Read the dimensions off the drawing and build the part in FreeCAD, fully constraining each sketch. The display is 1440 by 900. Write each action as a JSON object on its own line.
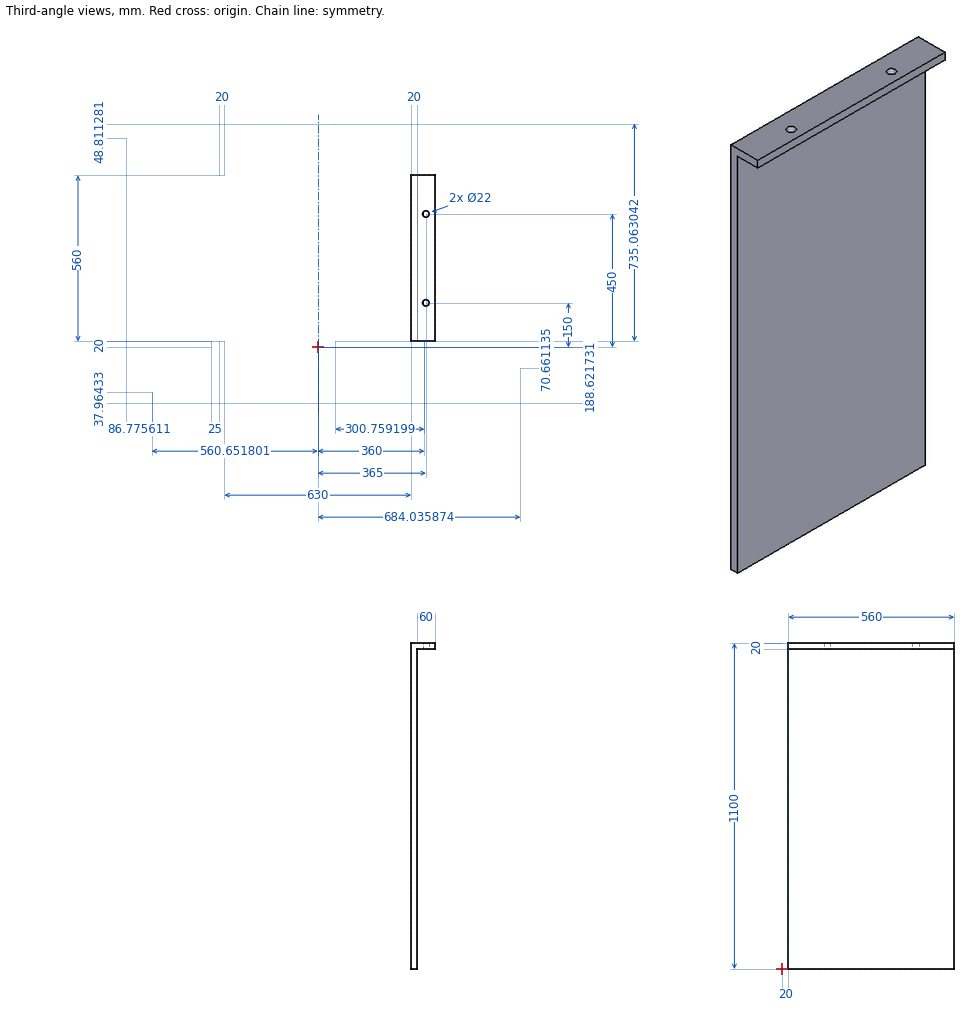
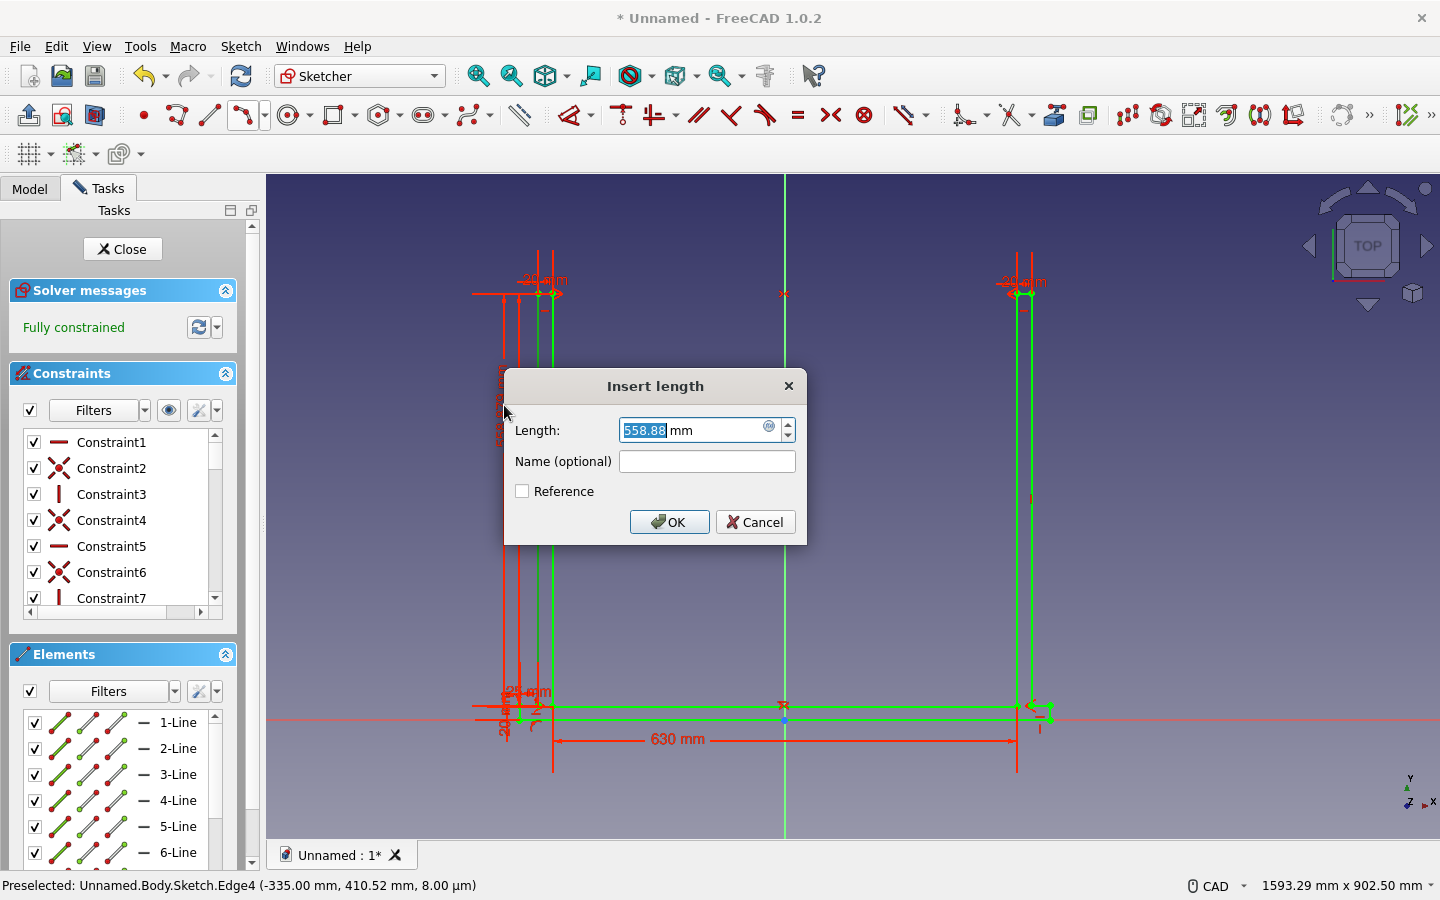
{"action": "type", "text": "560"}
{"action": "key", "text": "Return"}
{"action": "key", "text": "Escape"}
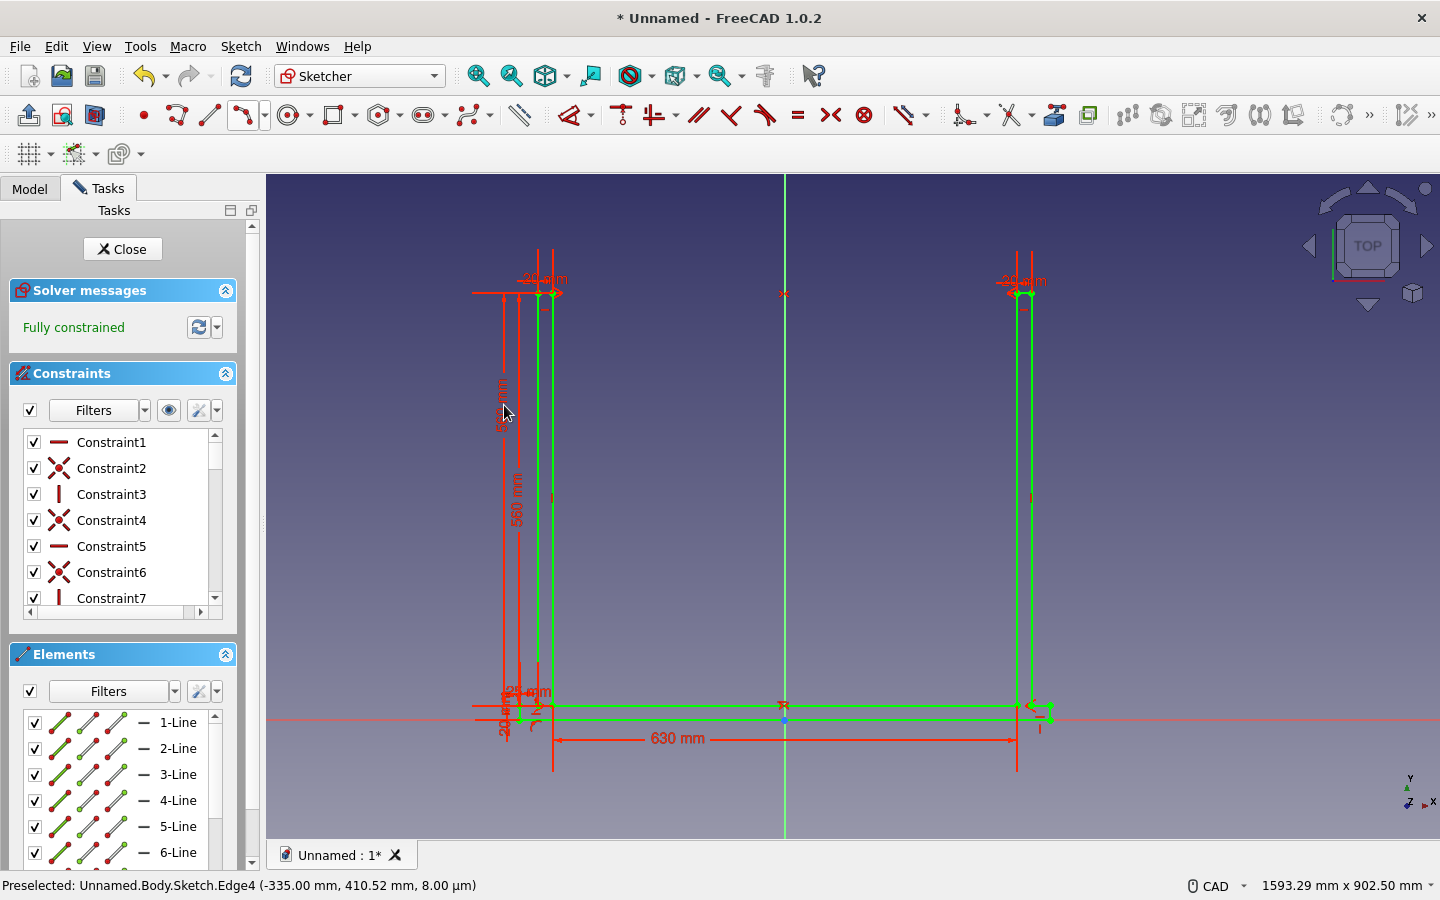
{"action": "left_click", "coordinate": [123, 249]}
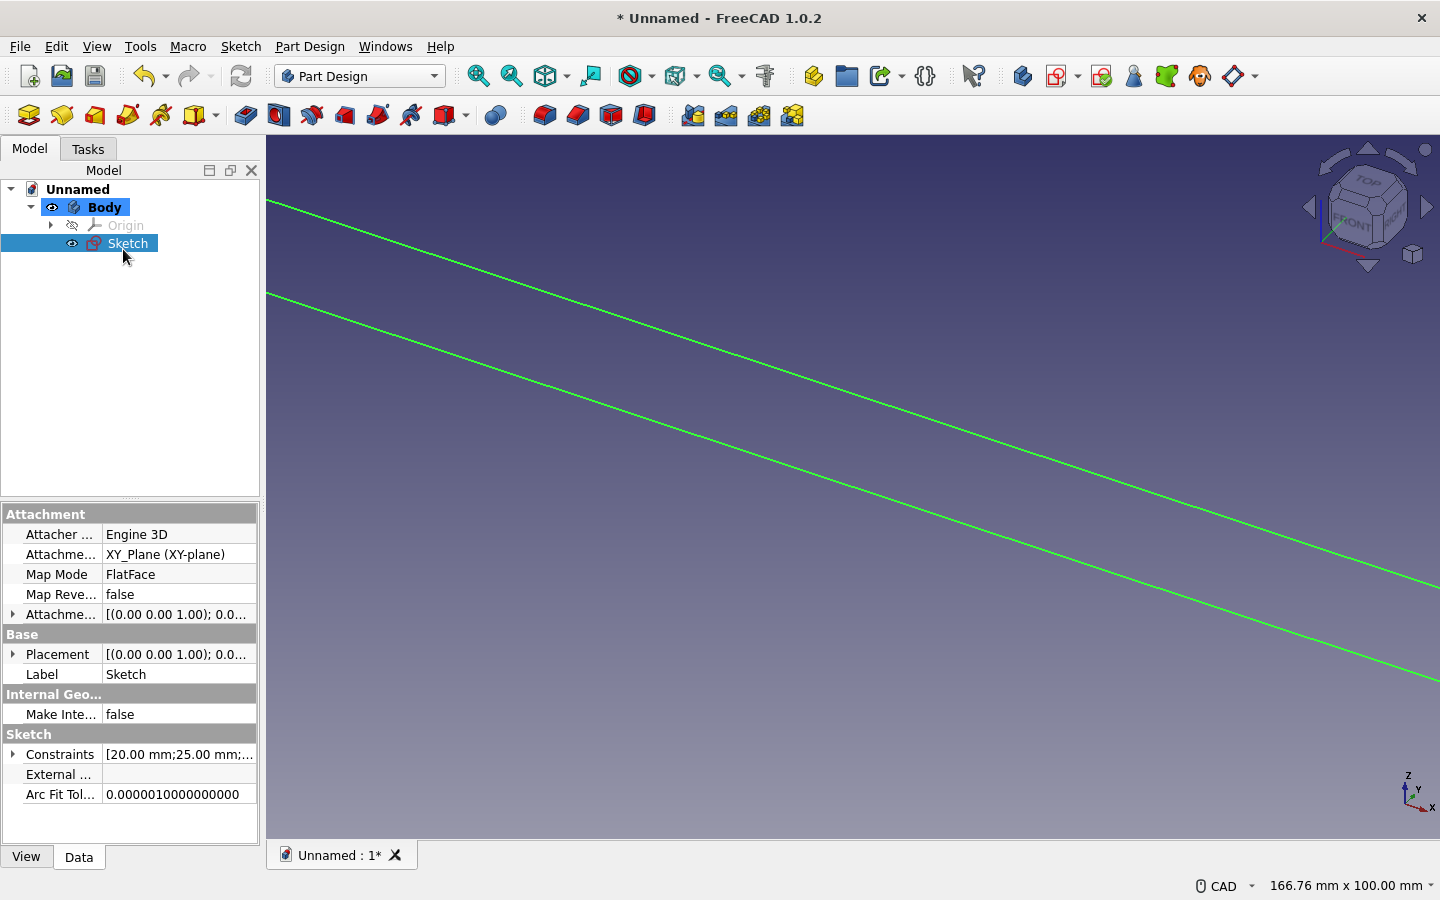
{"action": "left_click", "coordinate": [29, 116]}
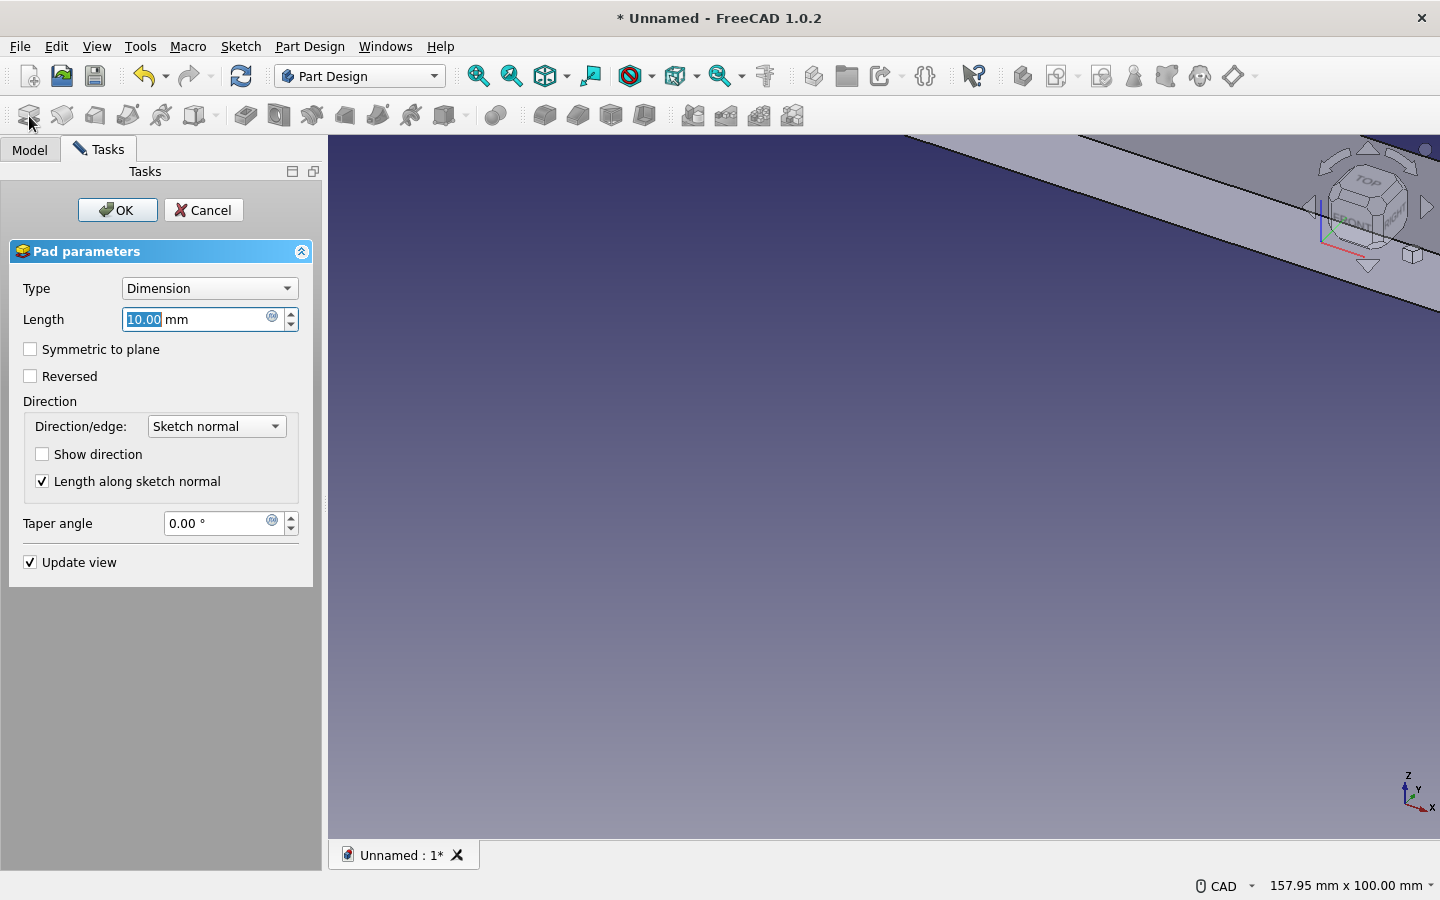
{"action": "type", "text": "1100"}
{"action": "key", "text": "Tab"}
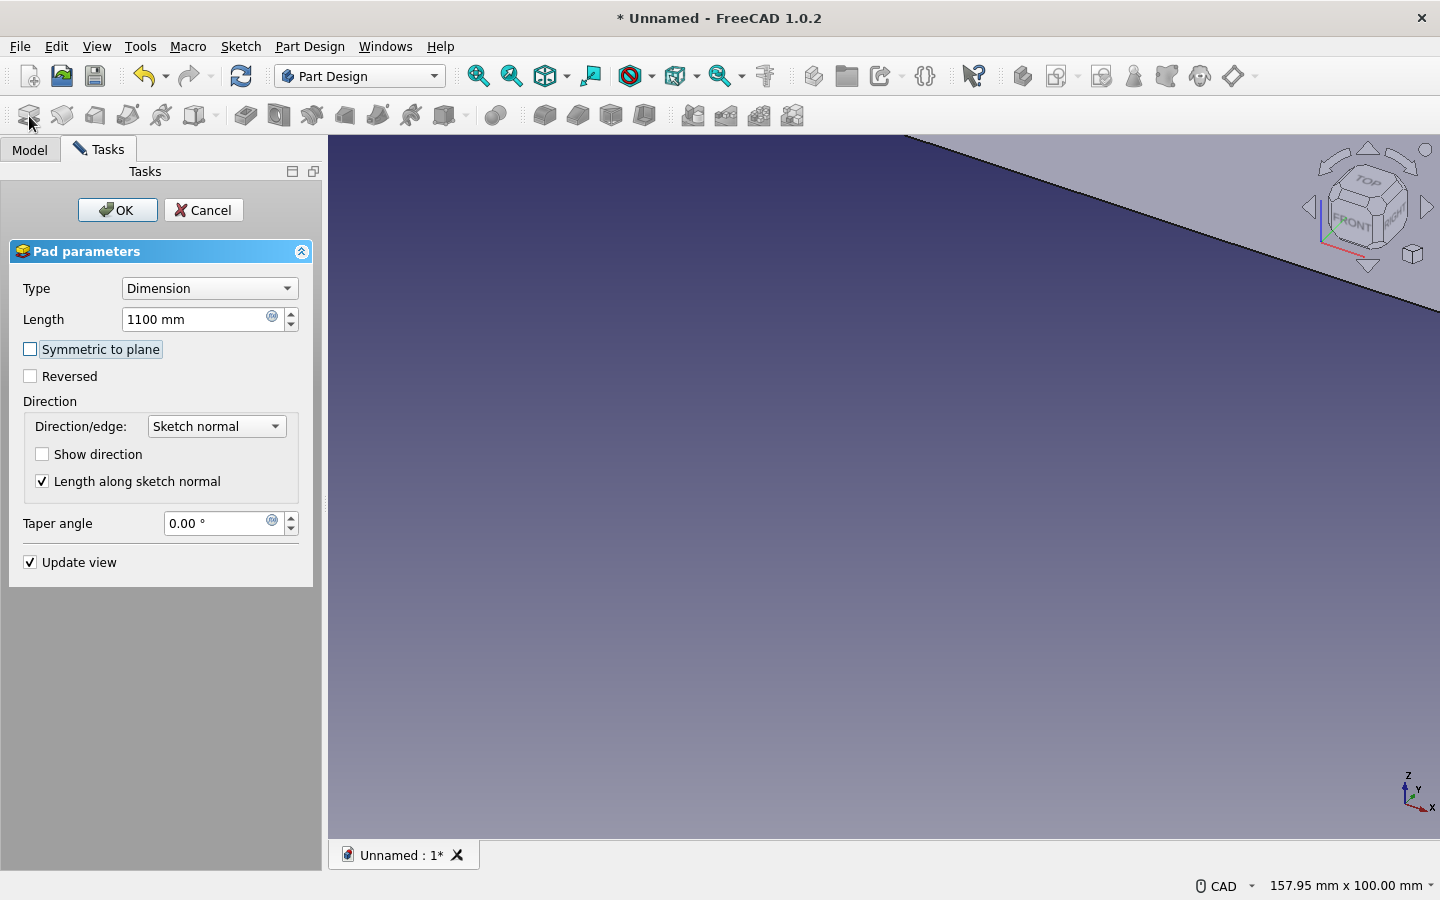
{"action": "left_click", "coordinate": [118, 210]}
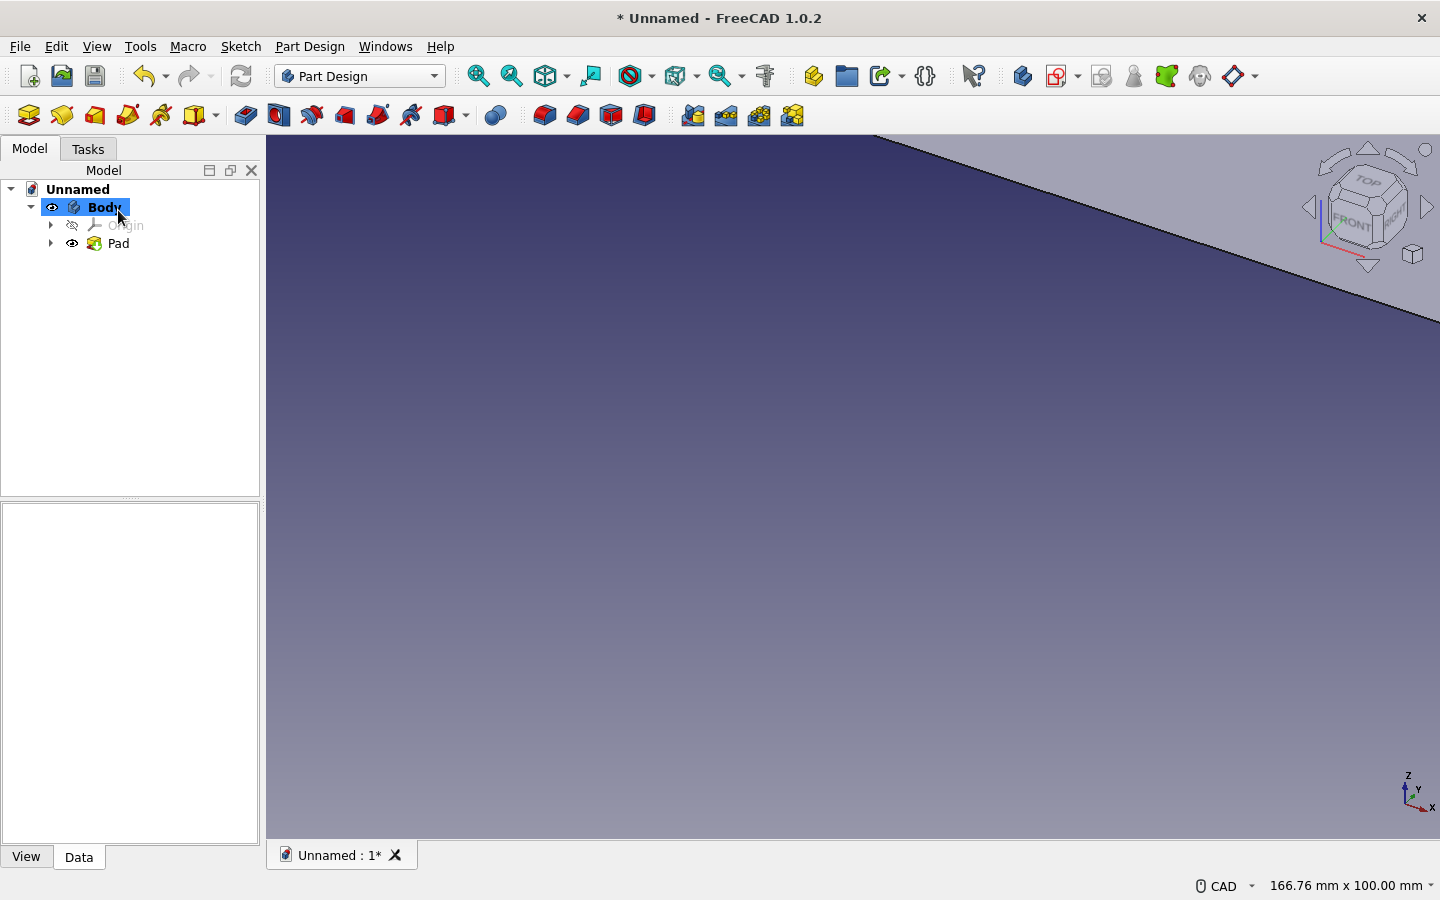
{"action": "left_click", "coordinate": [479, 76]}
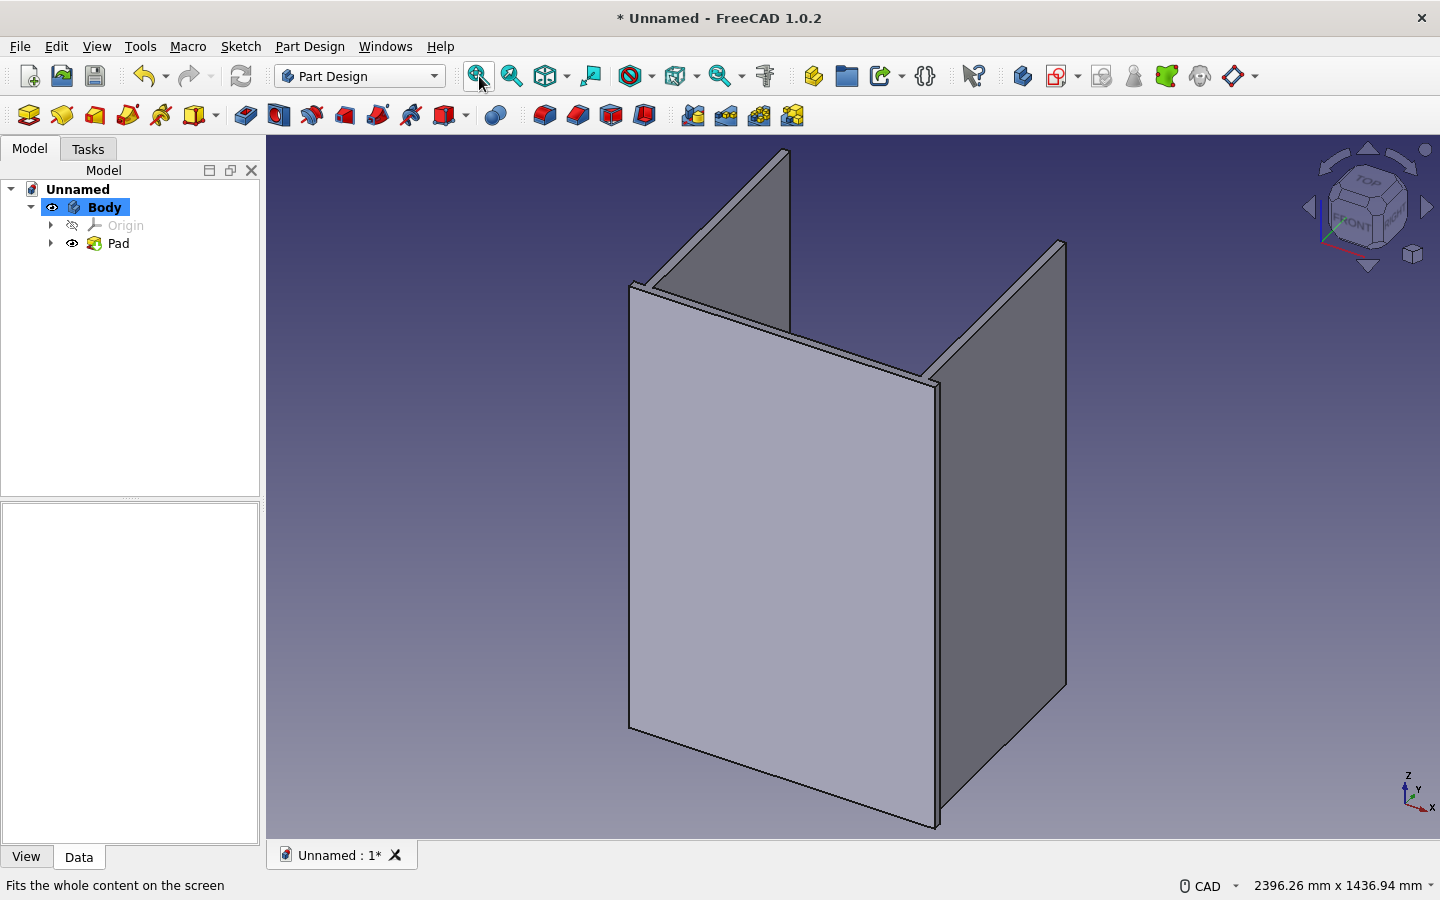
{"action": "left_click", "coordinate": [1056, 76]}